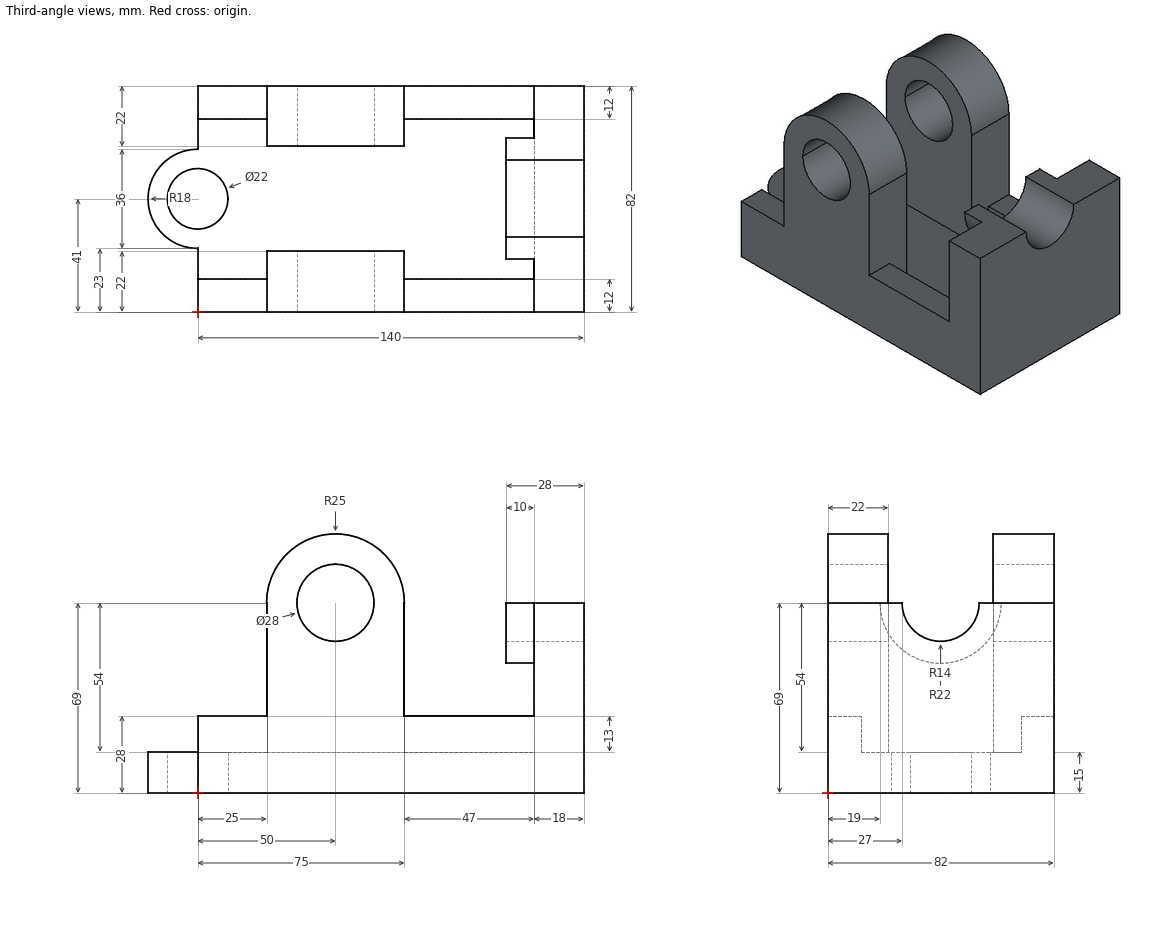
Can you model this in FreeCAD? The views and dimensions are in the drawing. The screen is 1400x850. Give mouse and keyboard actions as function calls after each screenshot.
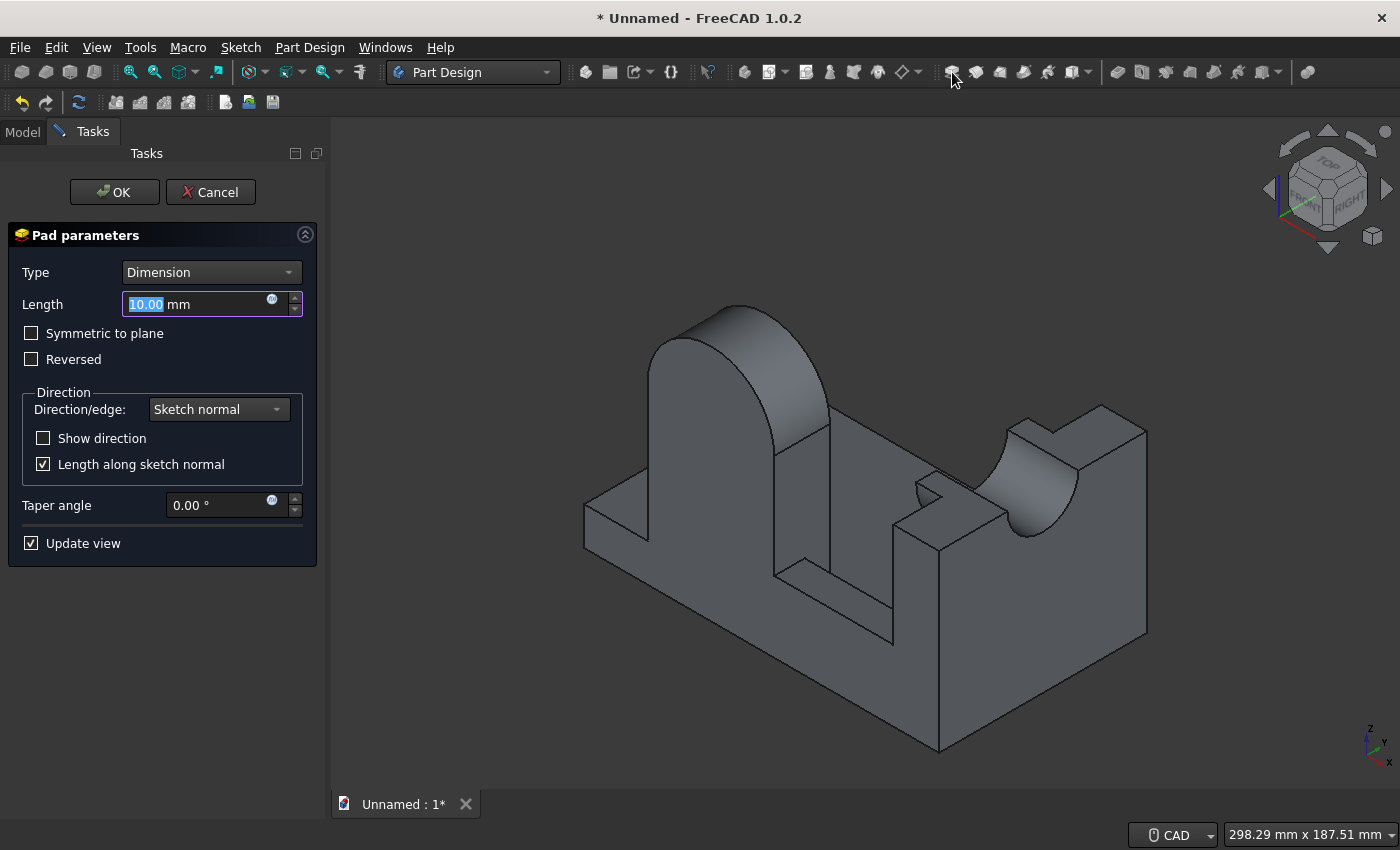
text(12)
key(Tab)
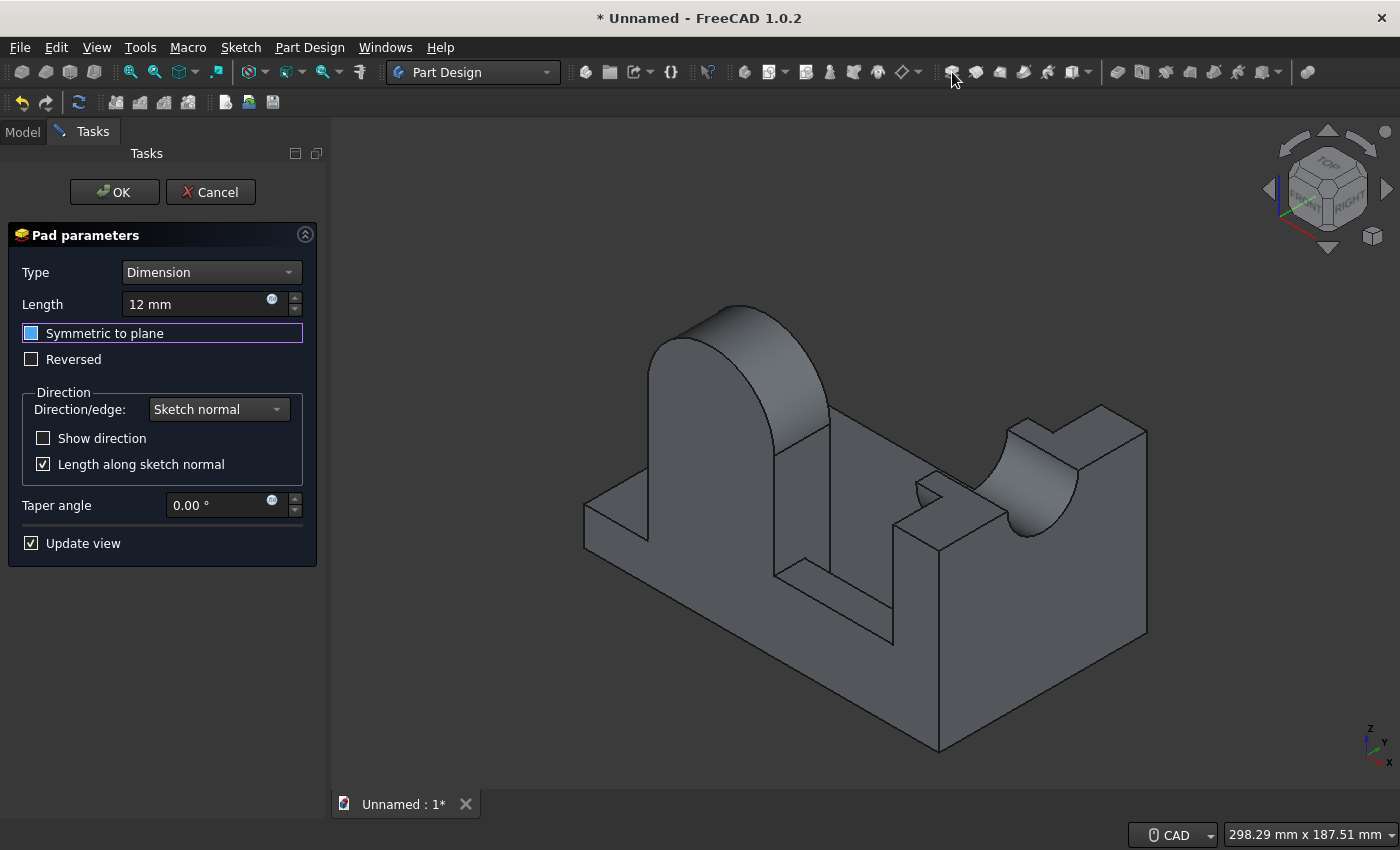
click(30, 359)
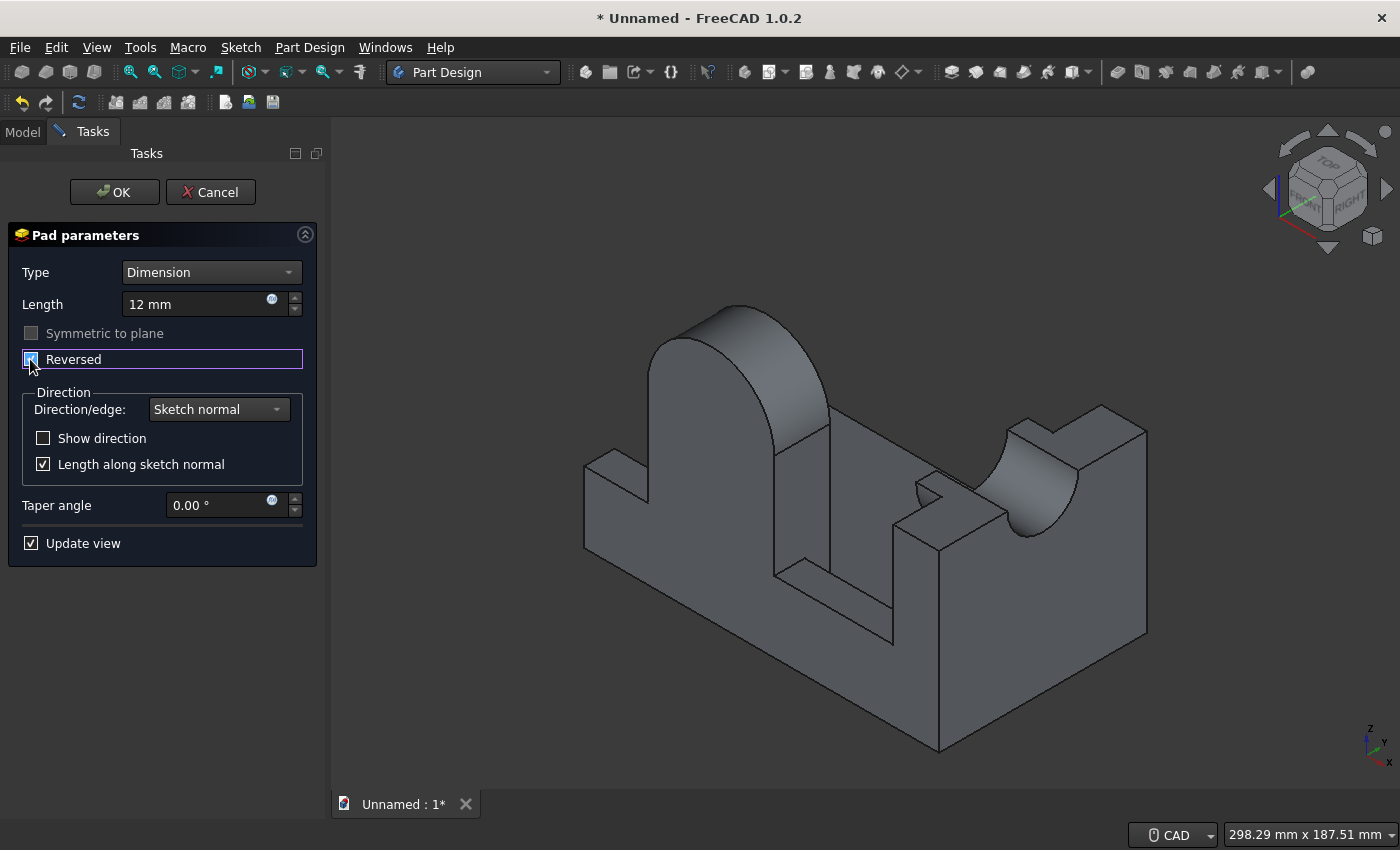
click(115, 192)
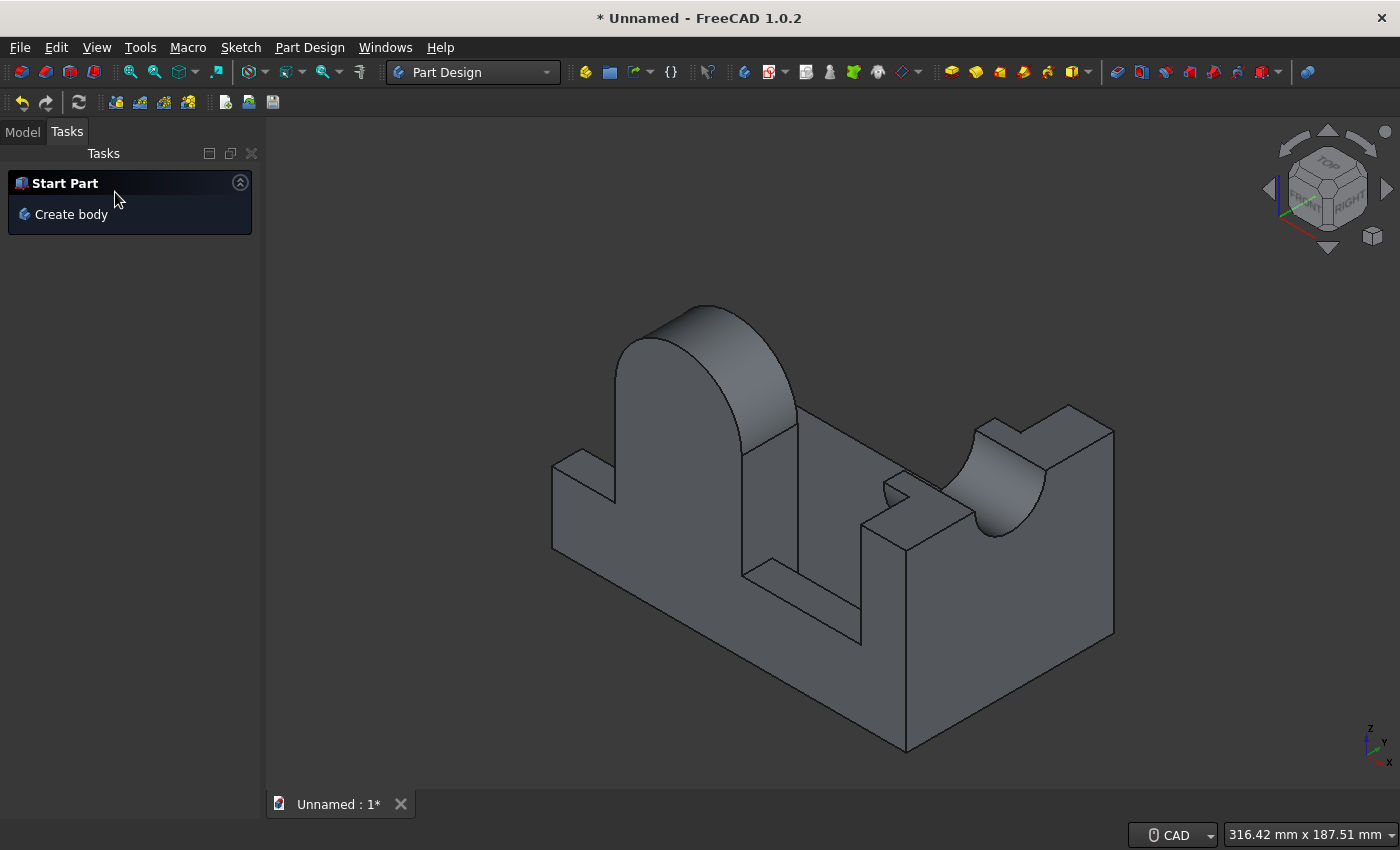
key(4)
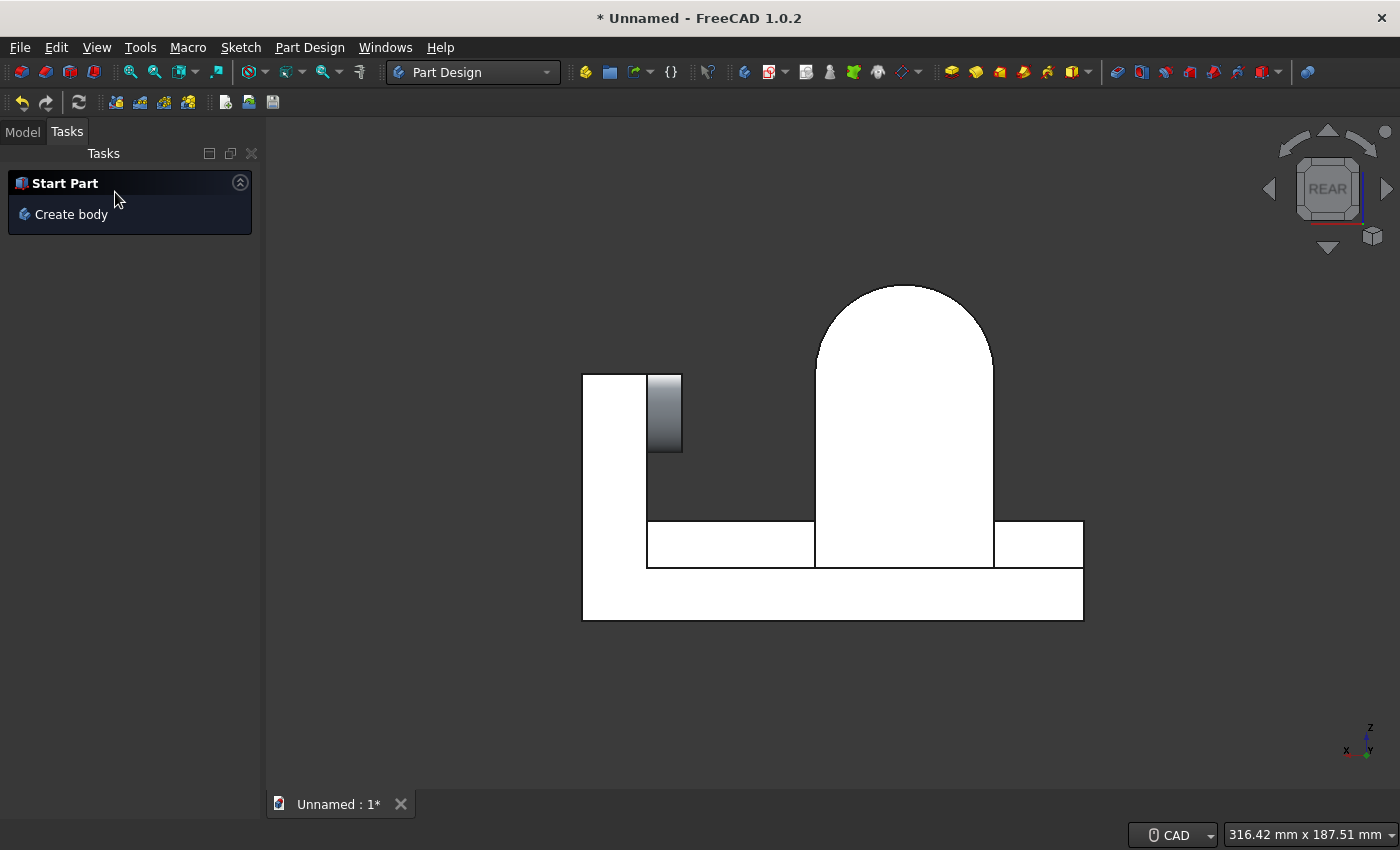
click(618, 567)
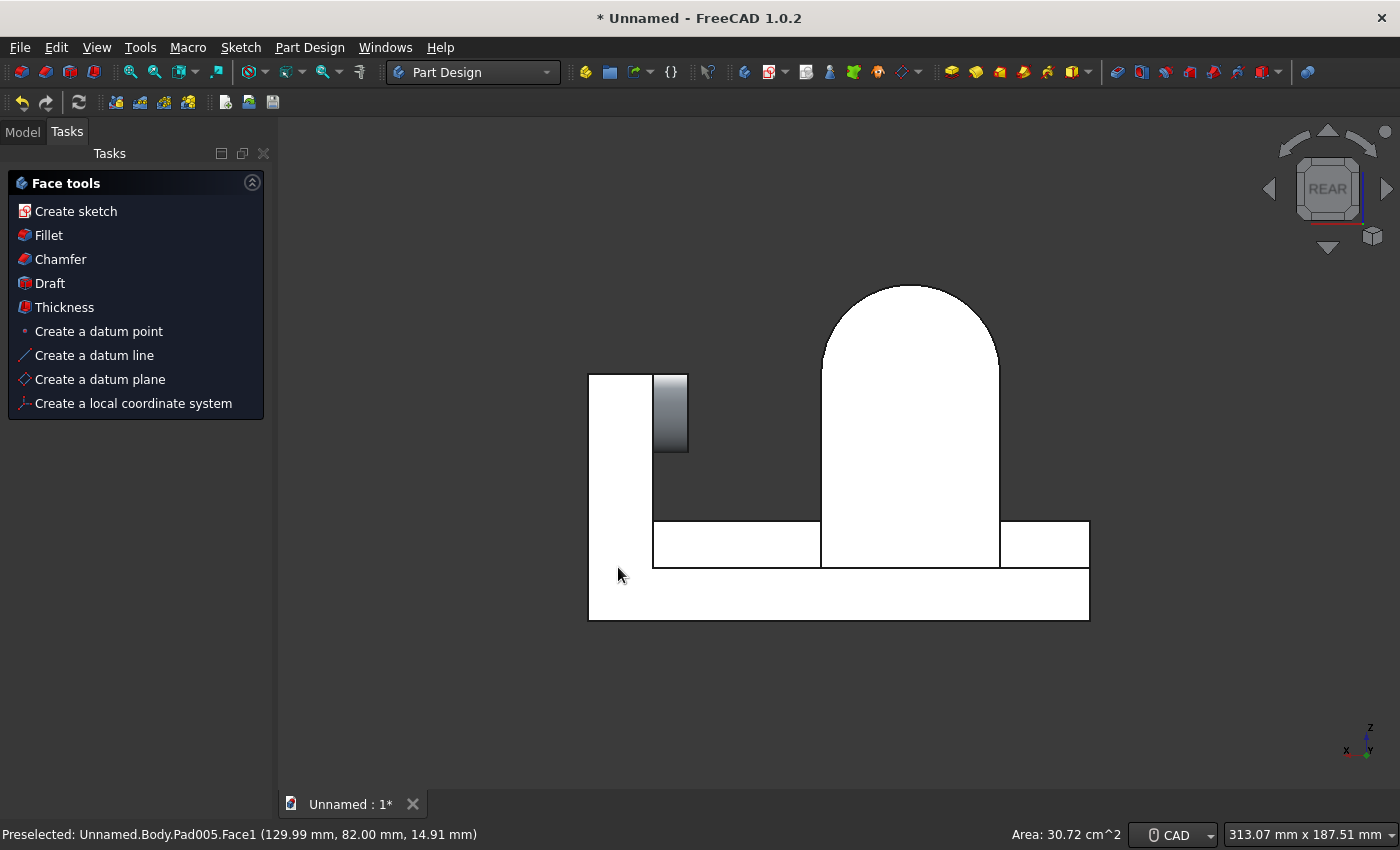
click(770, 72)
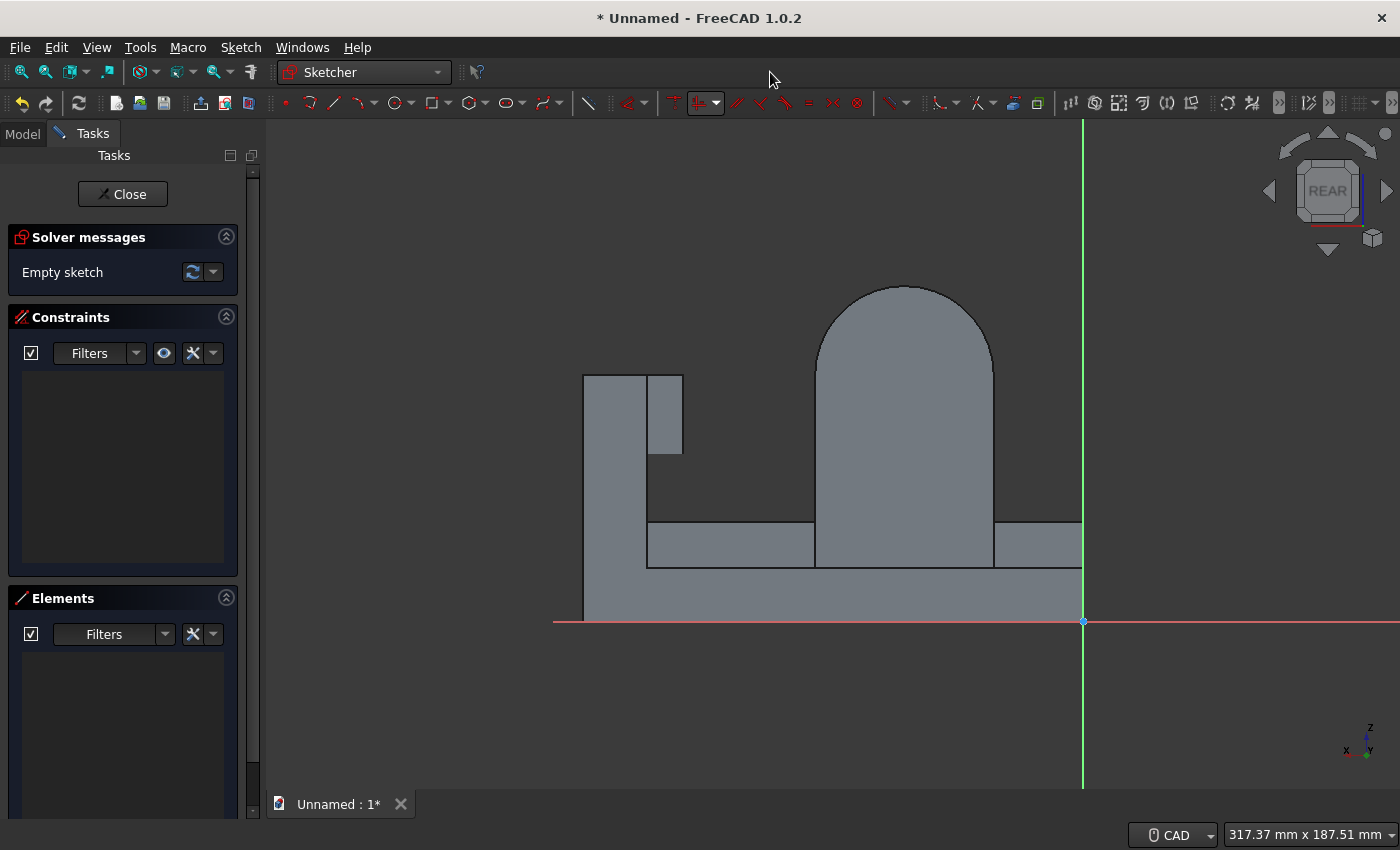
scroll(720, 575, up, 7)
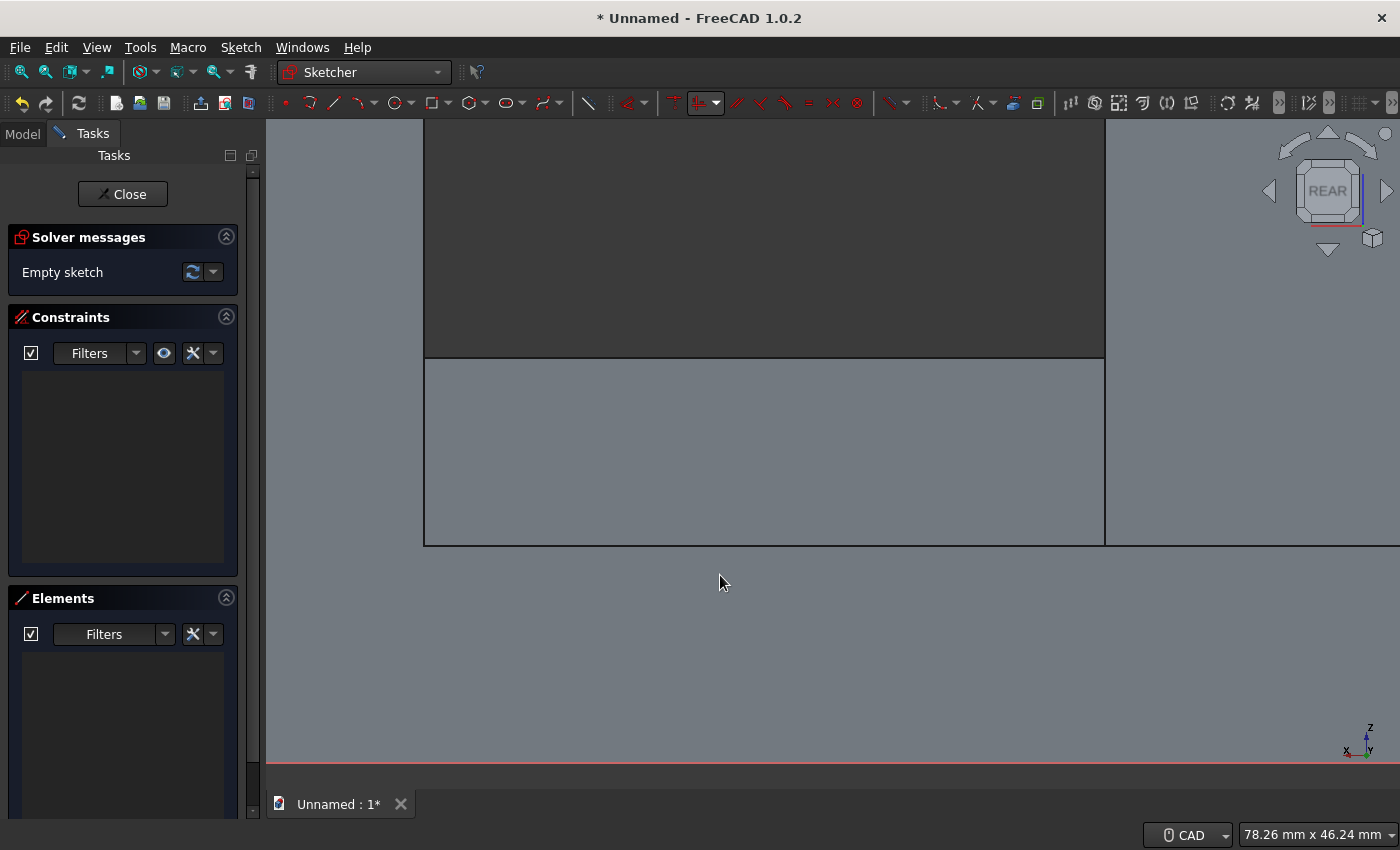
click(432, 104)